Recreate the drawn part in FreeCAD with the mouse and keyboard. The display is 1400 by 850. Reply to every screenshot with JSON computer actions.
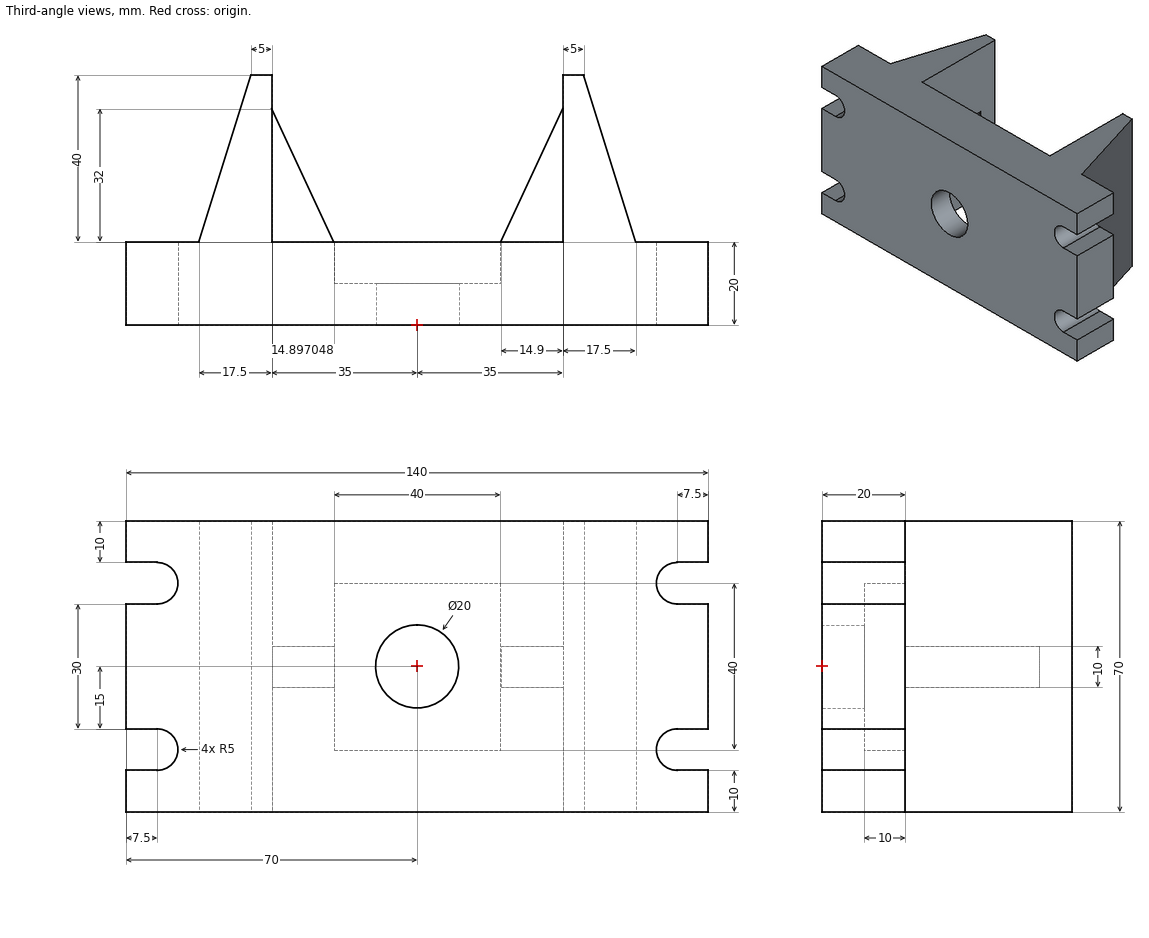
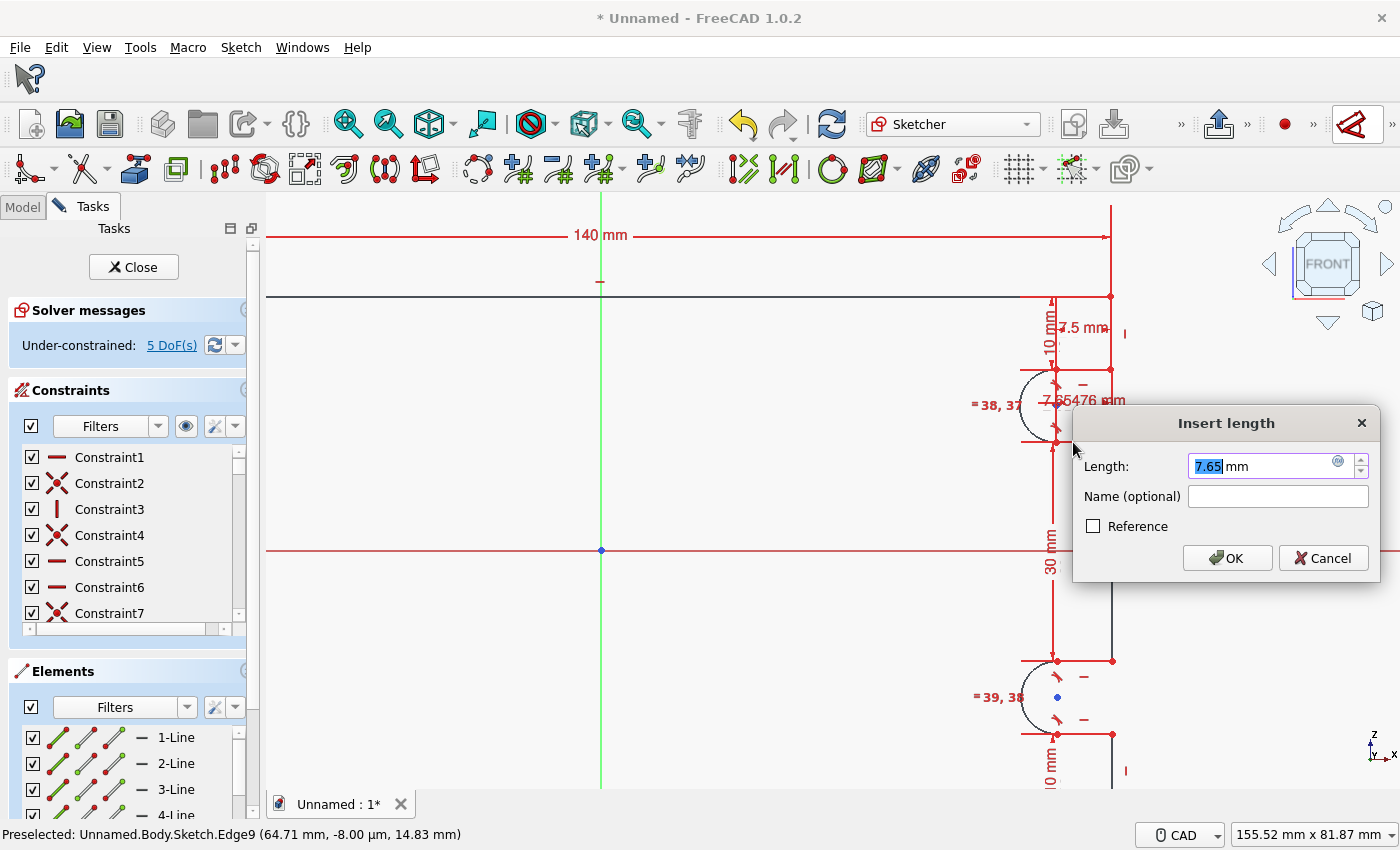
{"action": "type", "text": "7.5"}
{"action": "key", "text": "Return"}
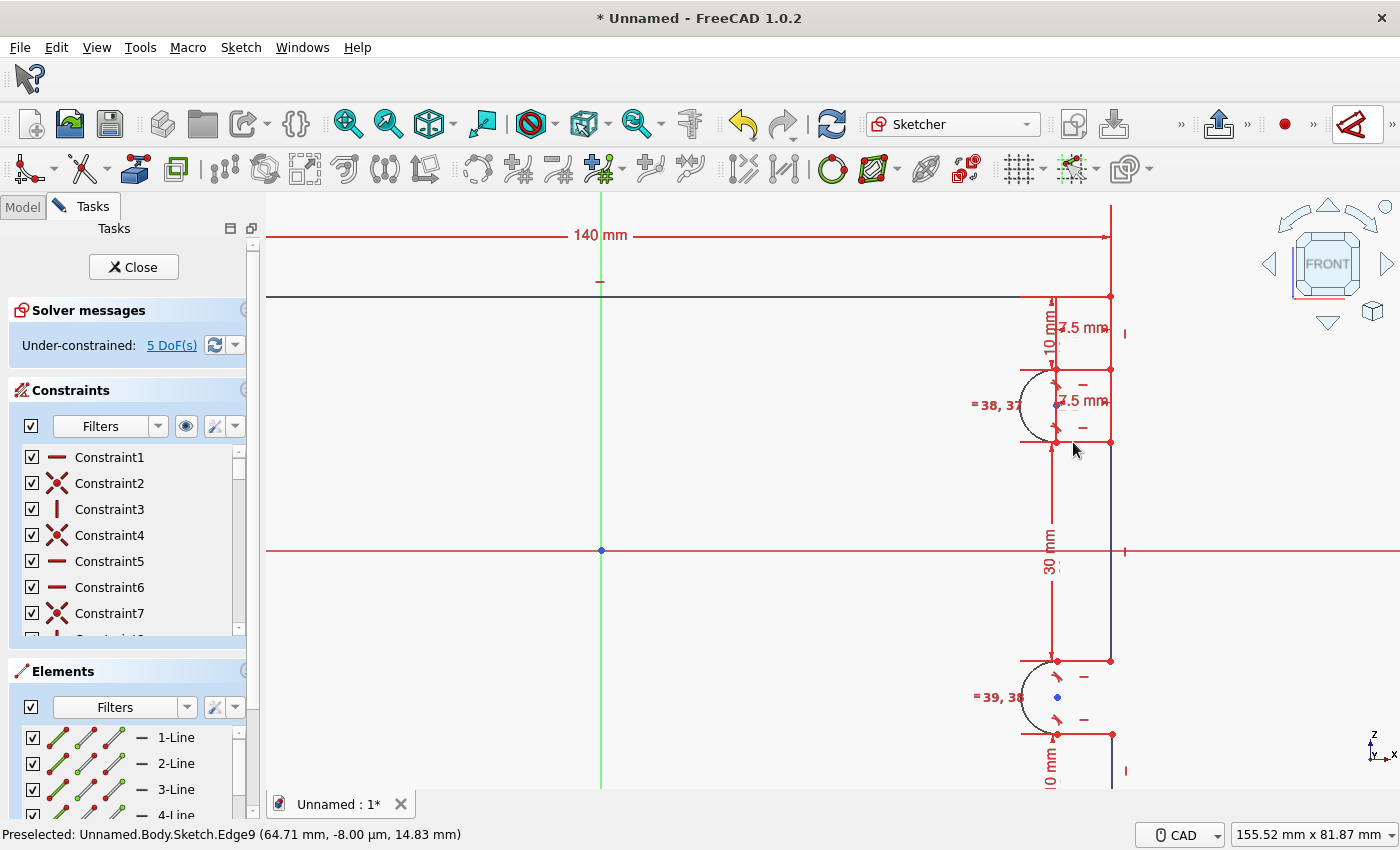
{"action": "left_click", "coordinate": [1095, 661]}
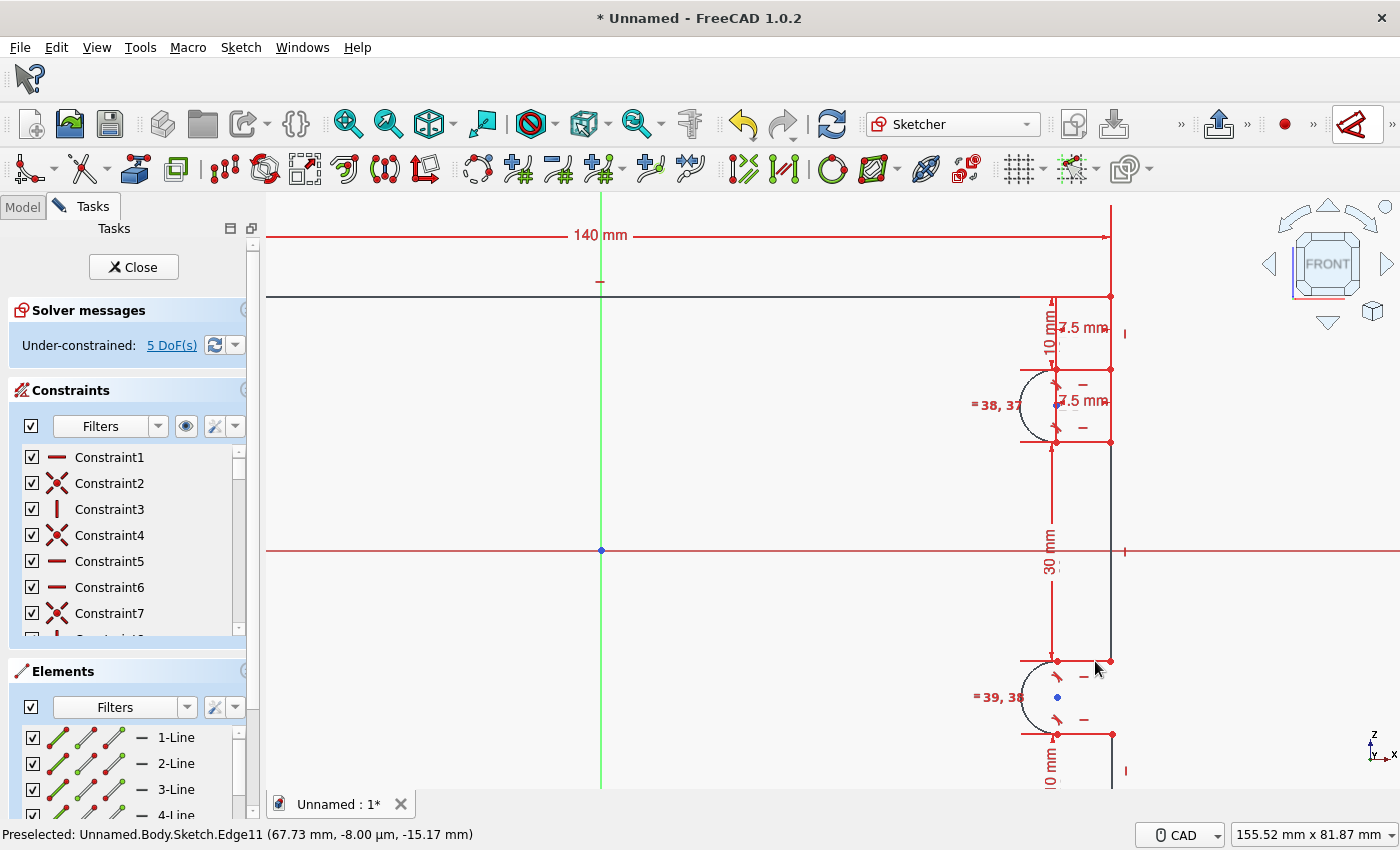
{"action": "left_click", "coordinate": [1378, 124]}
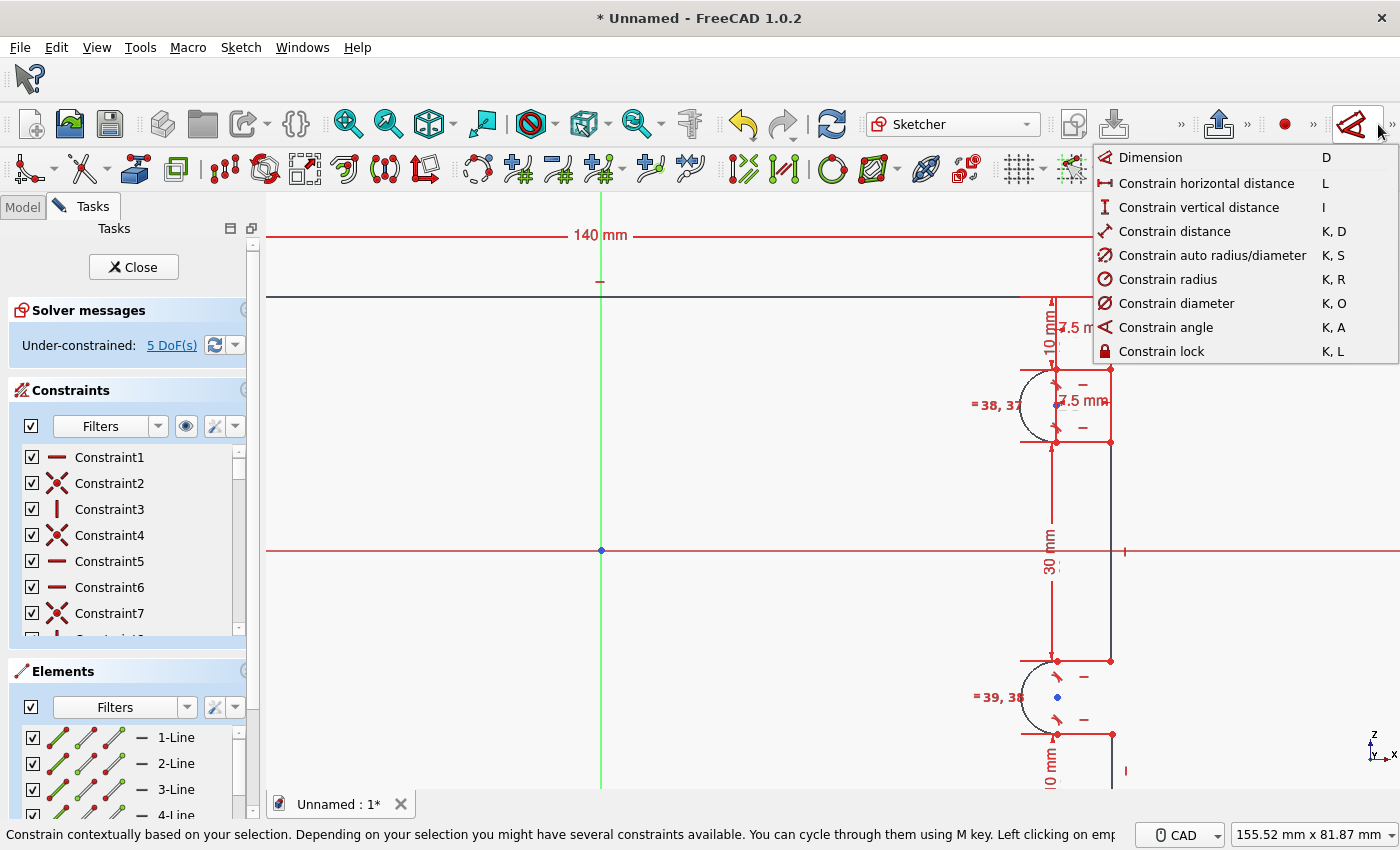
{"action": "left_click", "coordinate": [1246, 183]}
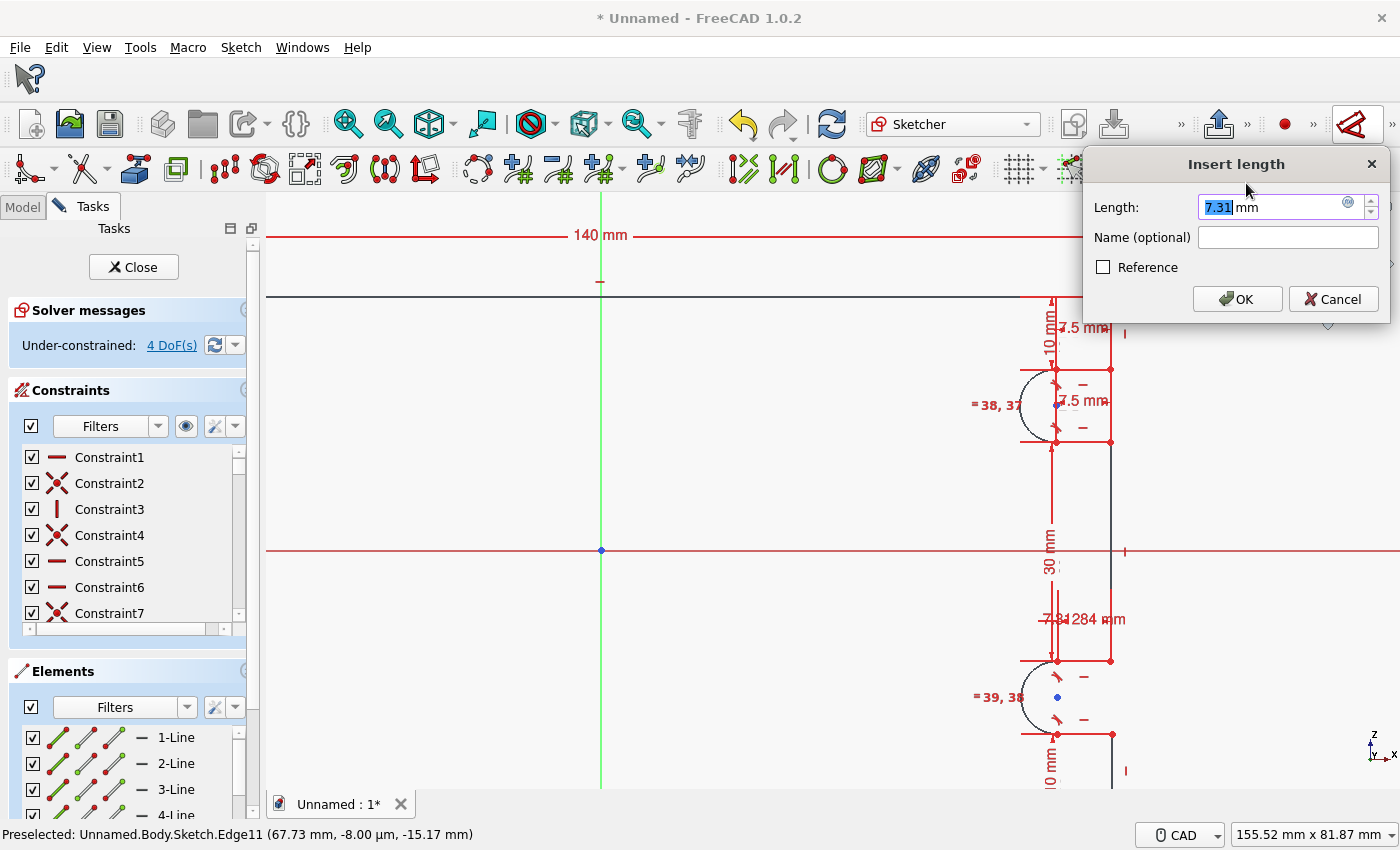
{"action": "type", "text": "7.5"}
{"action": "key", "text": "Return"}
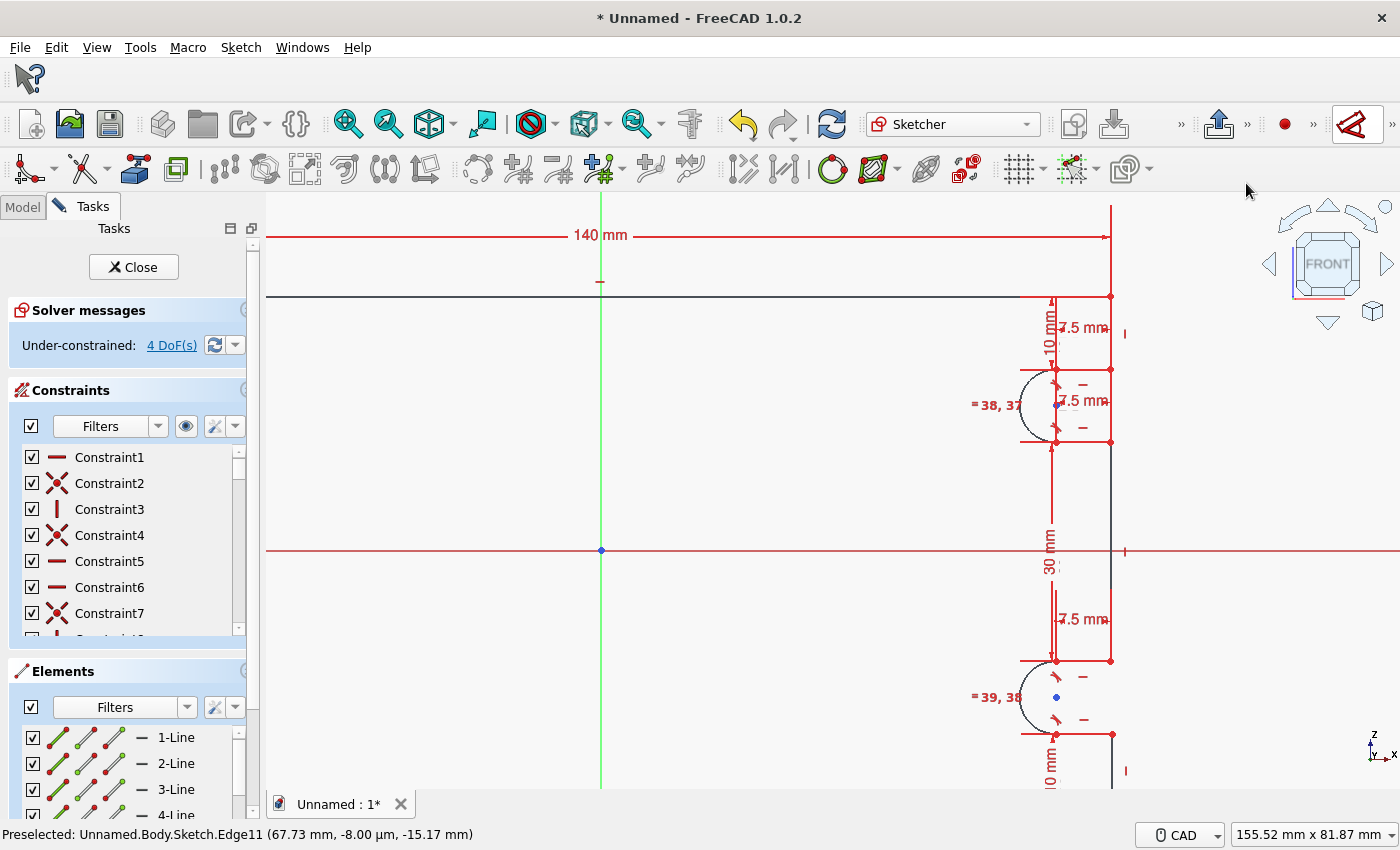
{"action": "left_click", "coordinate": [1073, 734]}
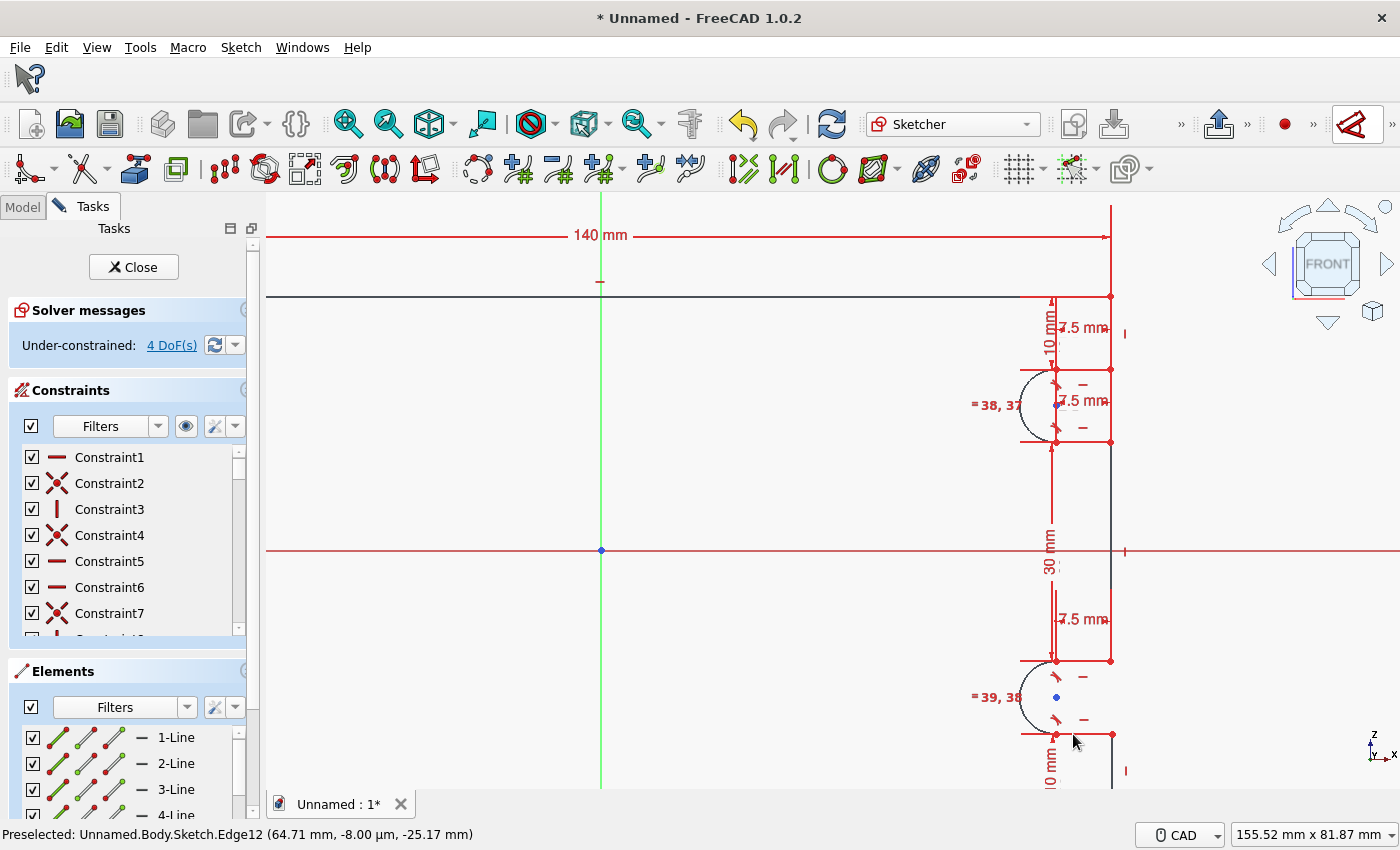
{"action": "key", "text": "l"}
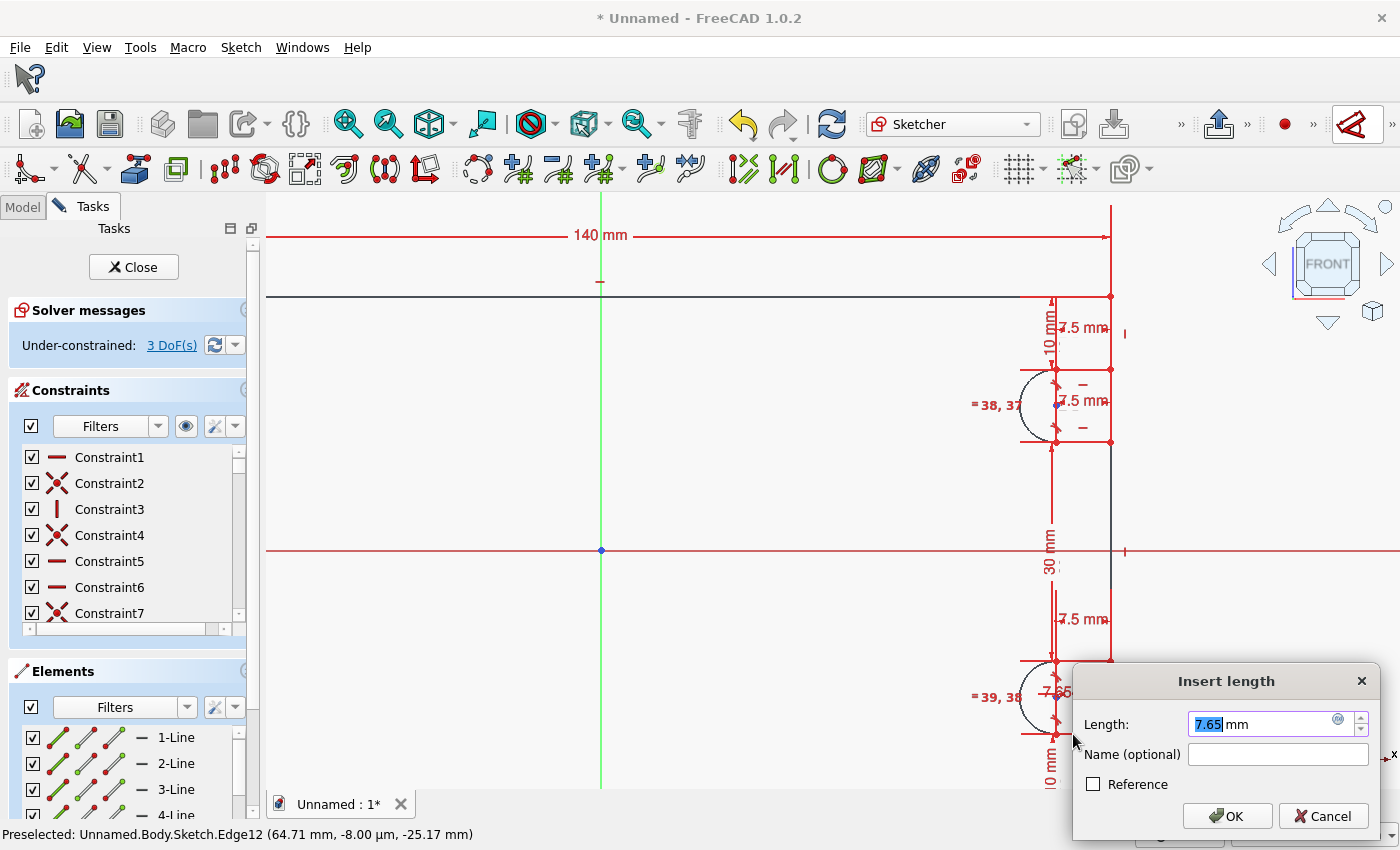
{"action": "type", "text": "7.5"}
{"action": "key", "text": "Return"}